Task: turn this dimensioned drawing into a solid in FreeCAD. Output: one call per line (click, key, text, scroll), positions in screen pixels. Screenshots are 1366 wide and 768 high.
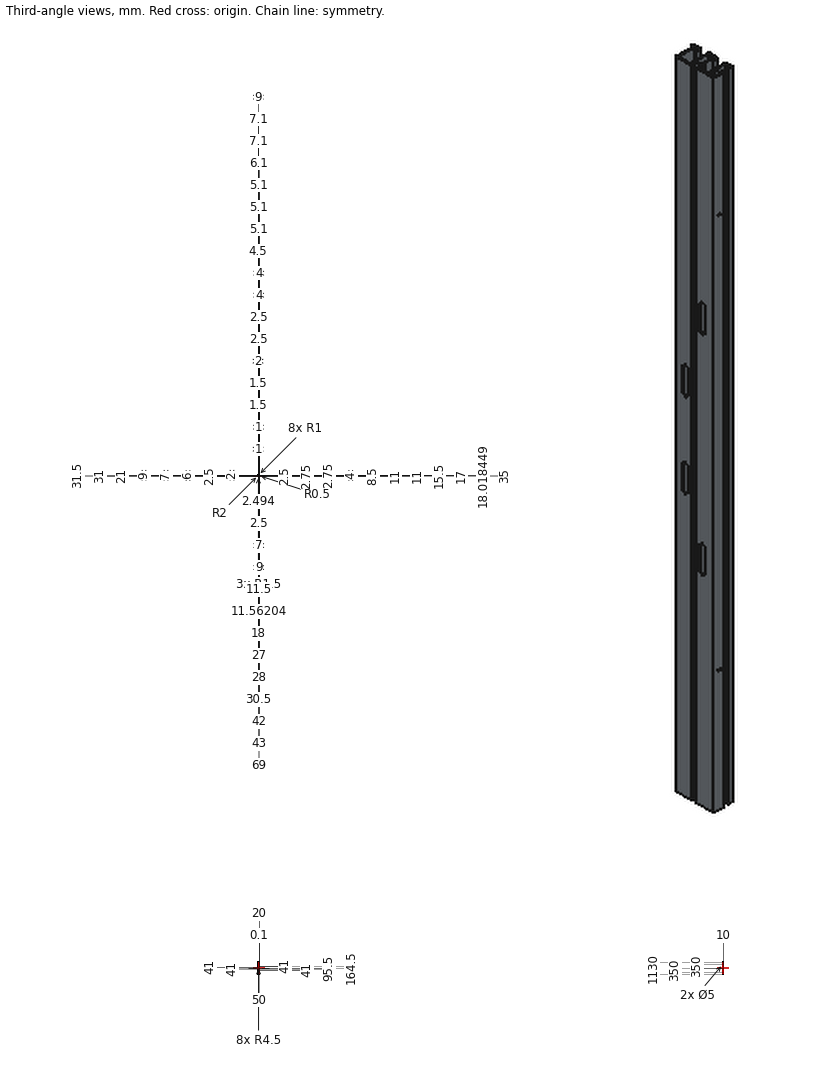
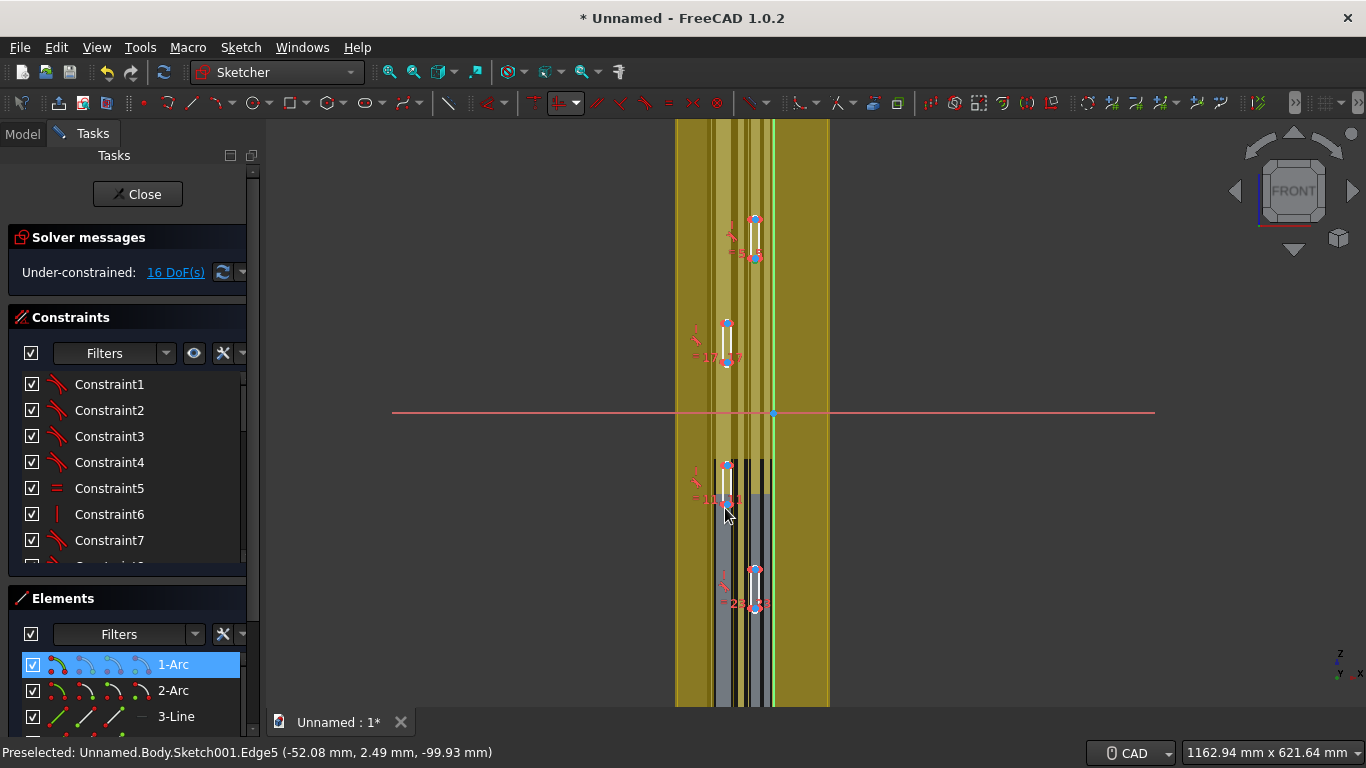
scroll(725, 366, up, 7)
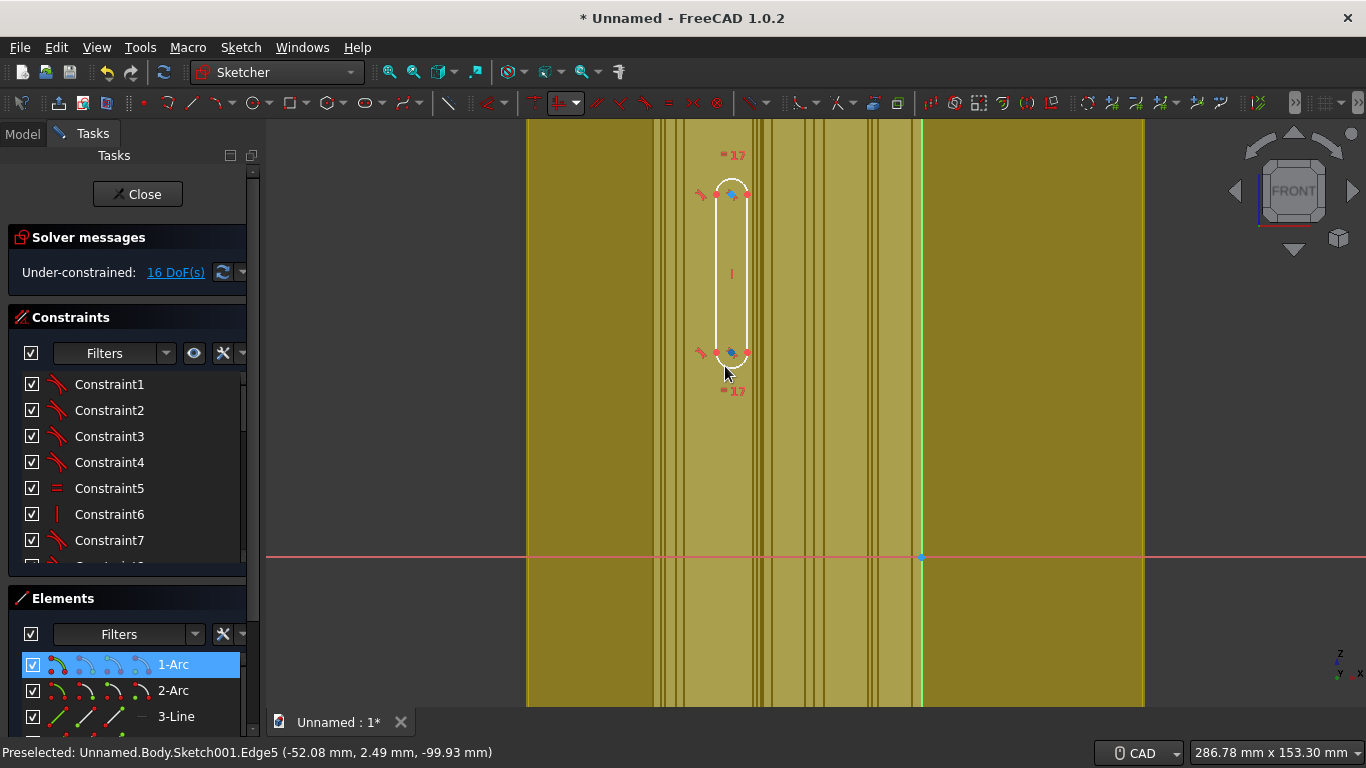
click(723, 365)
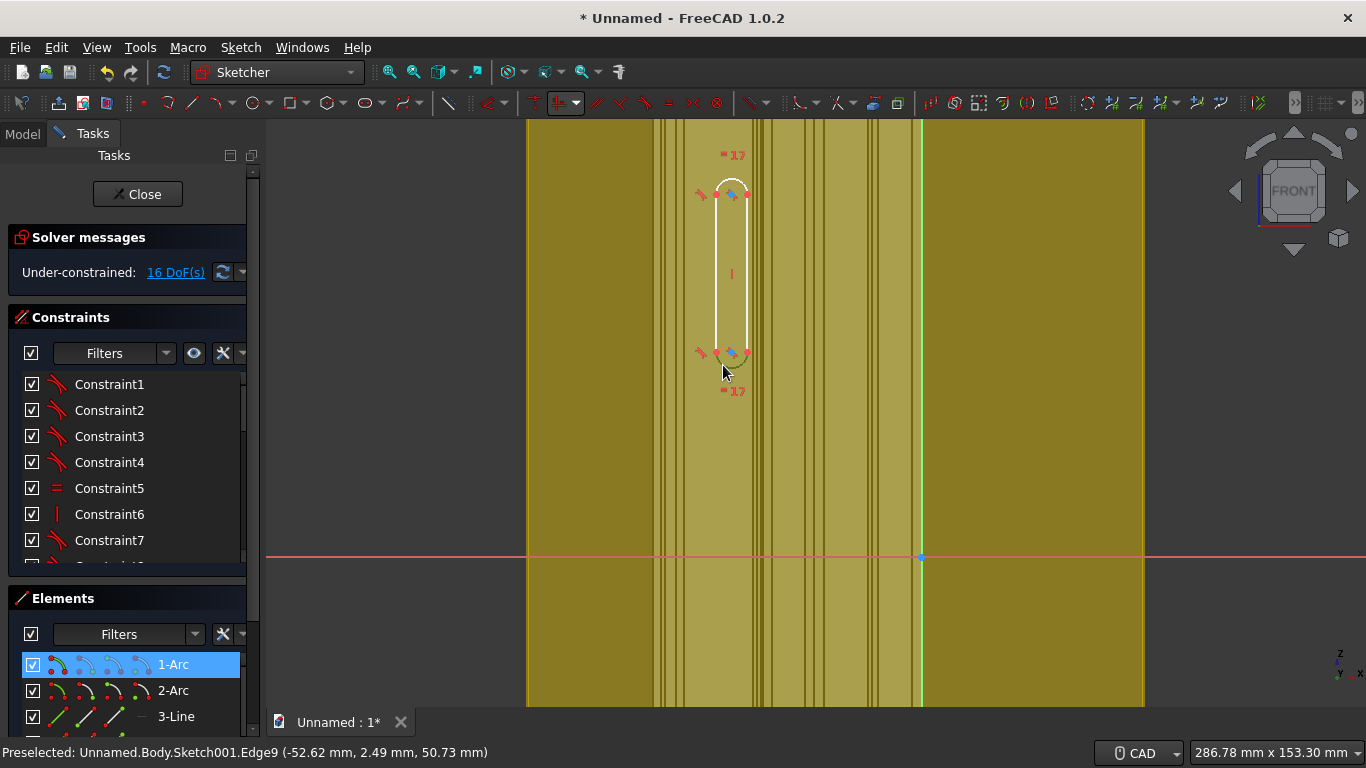
scroll(725, 366, down, 7)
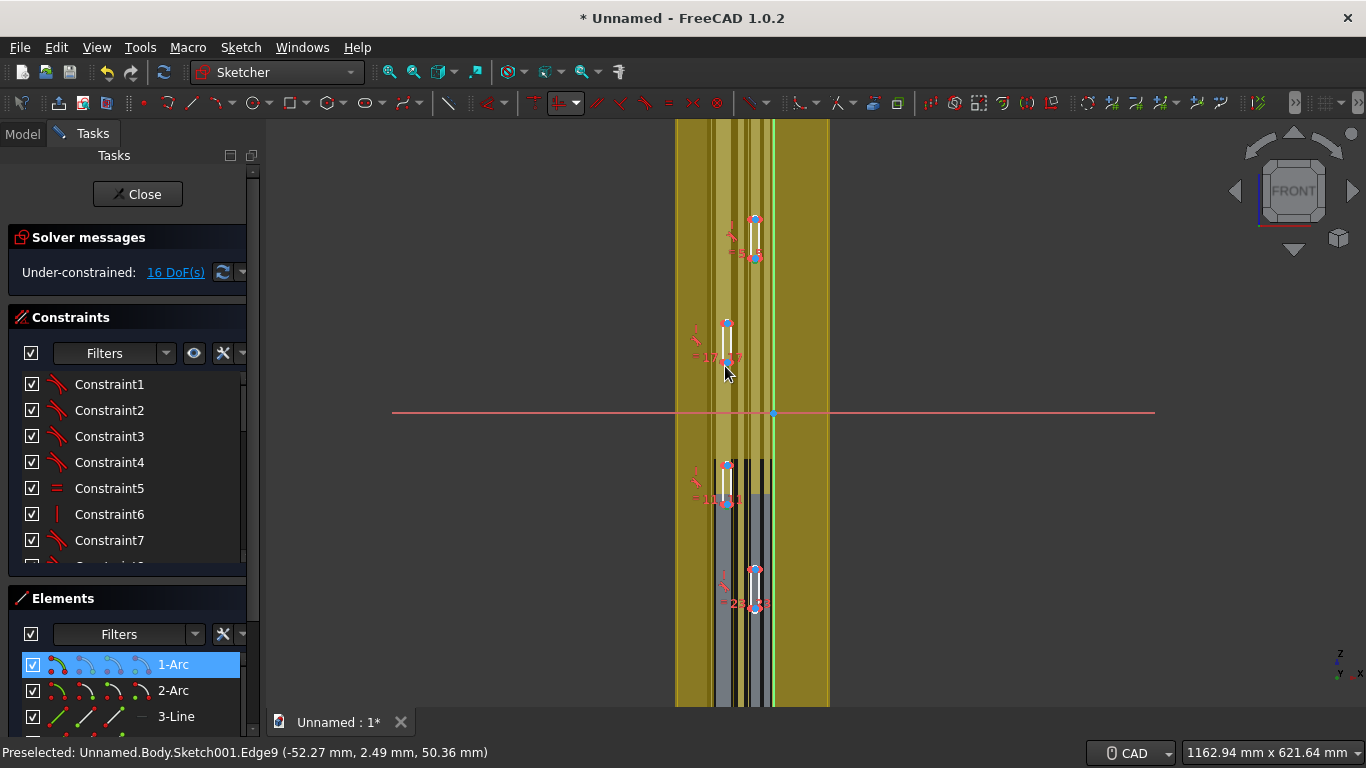
scroll(753, 612, up, 7)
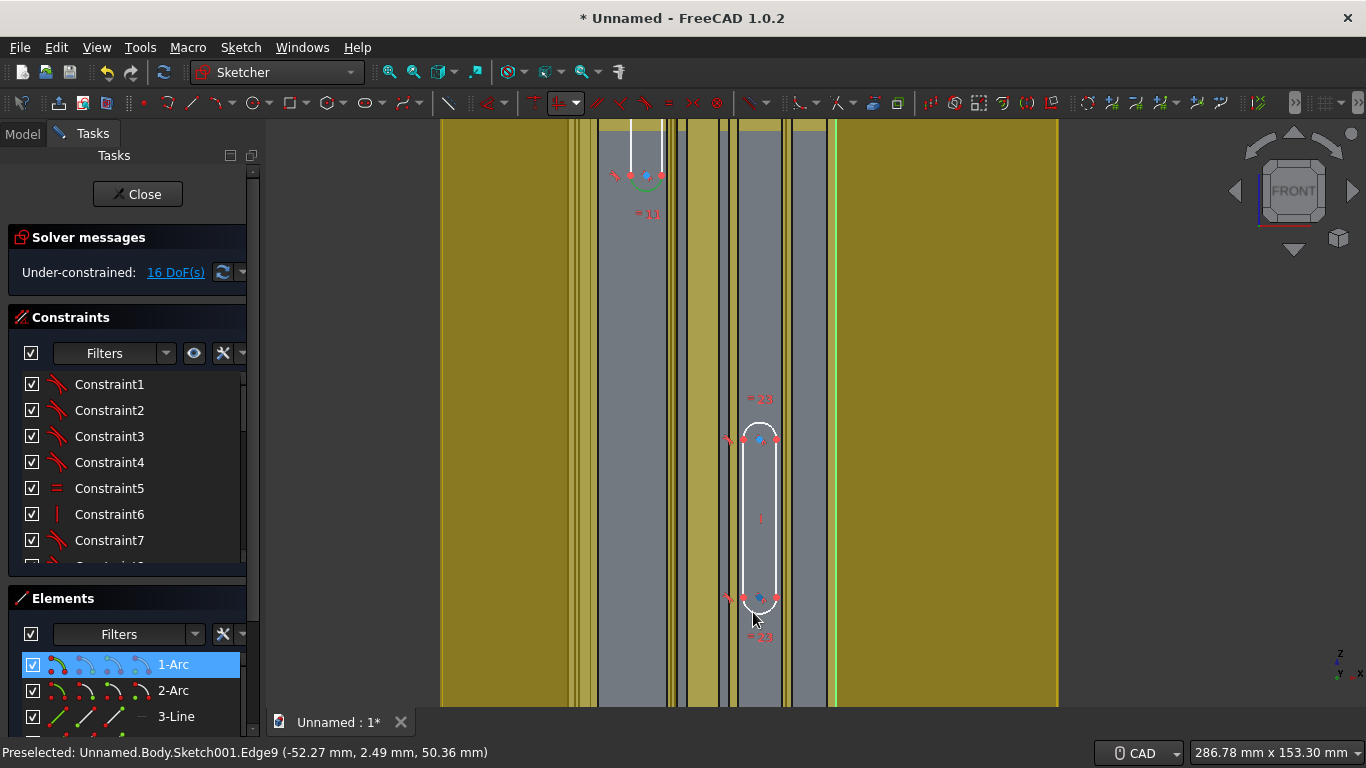
click(750, 611)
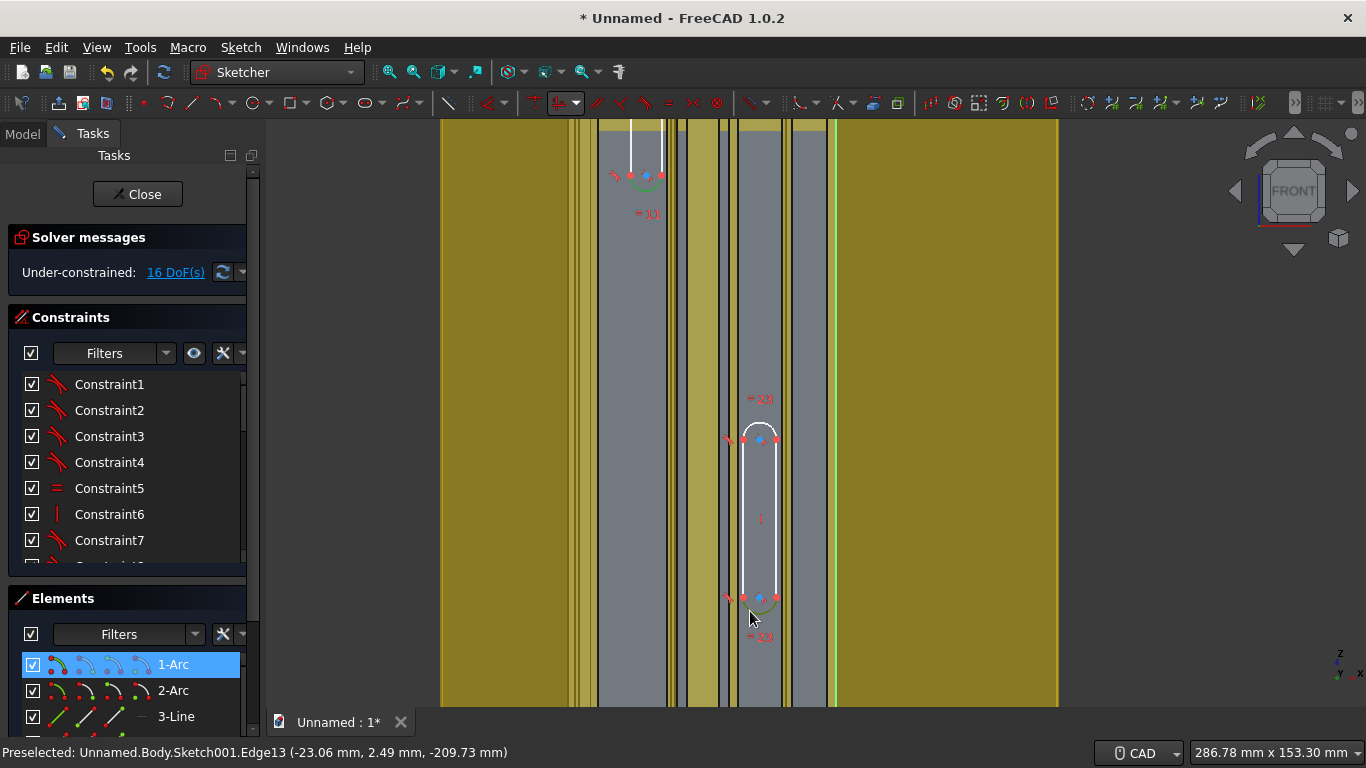
click(670, 104)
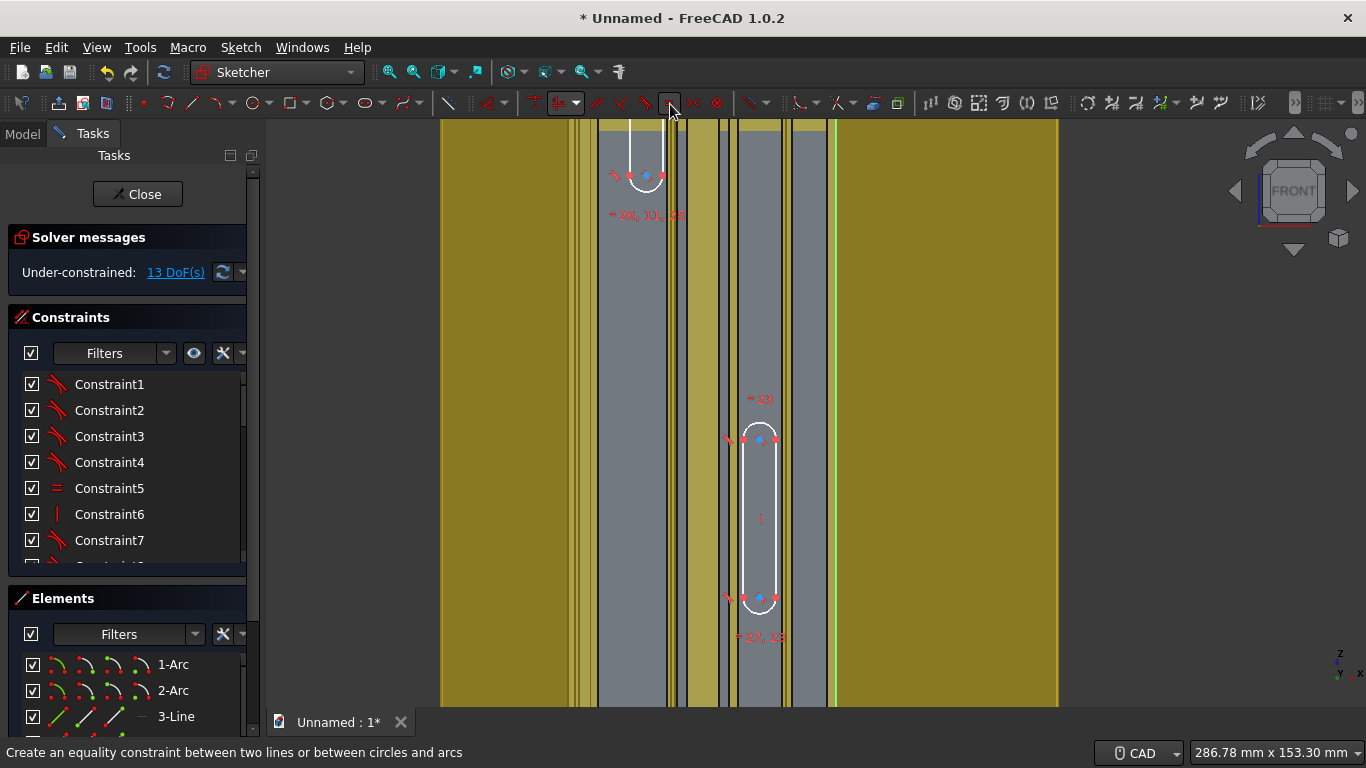
scroll(753, 612, down, 7)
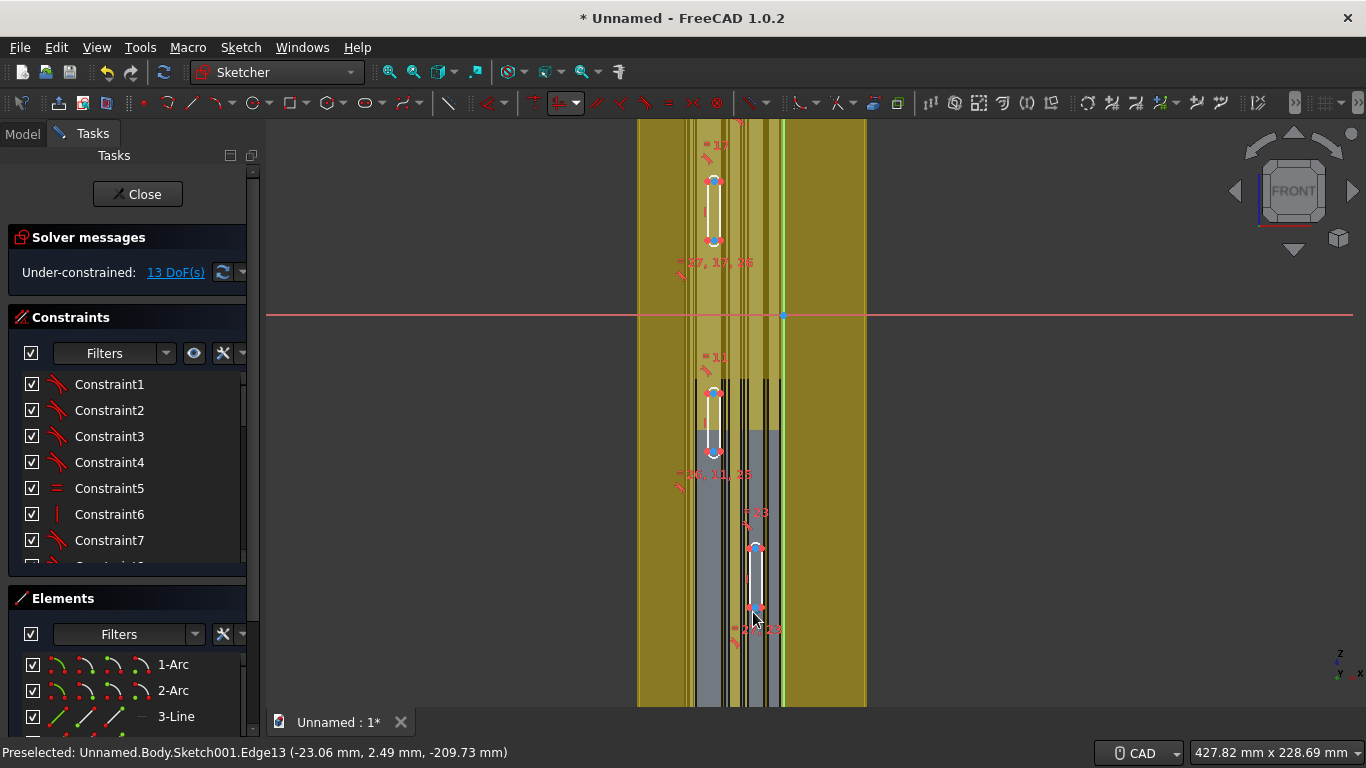
scroll(727, 466, up, 6)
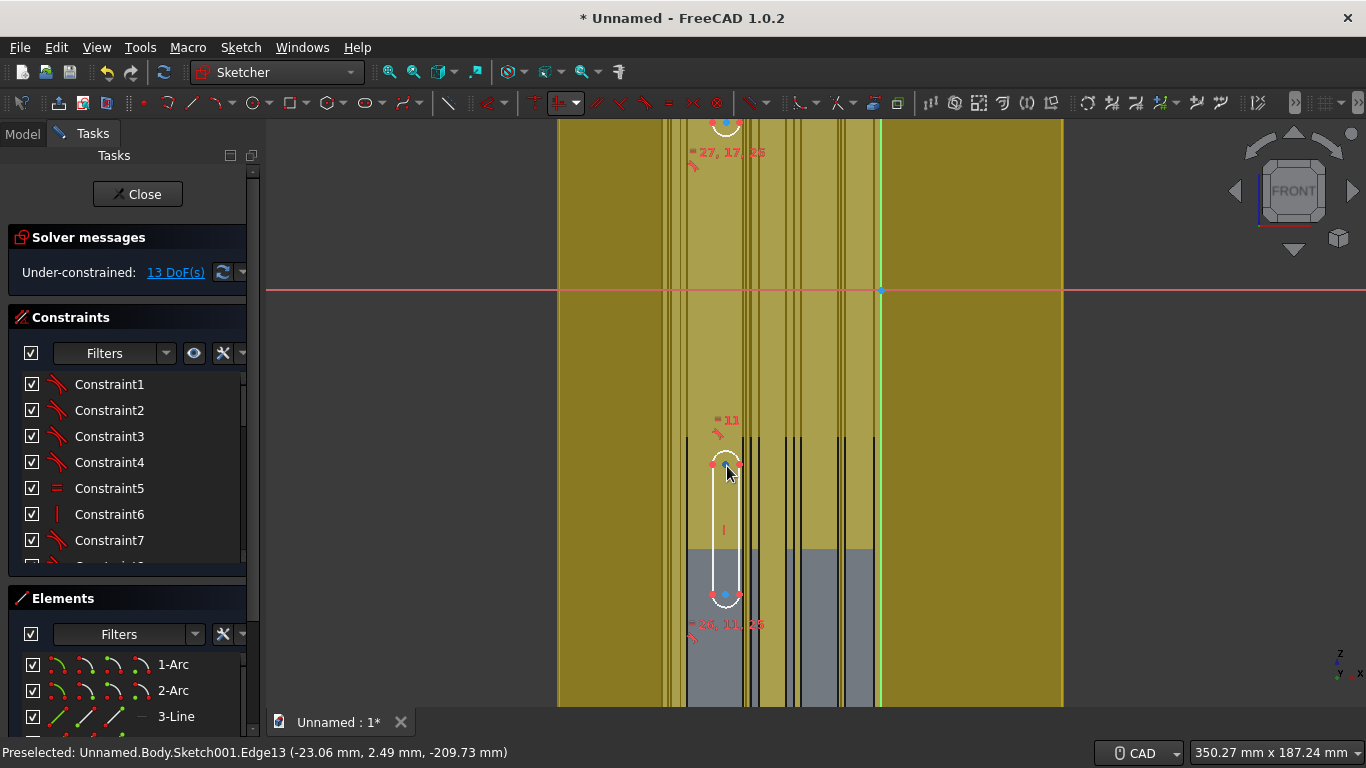
click(726, 465)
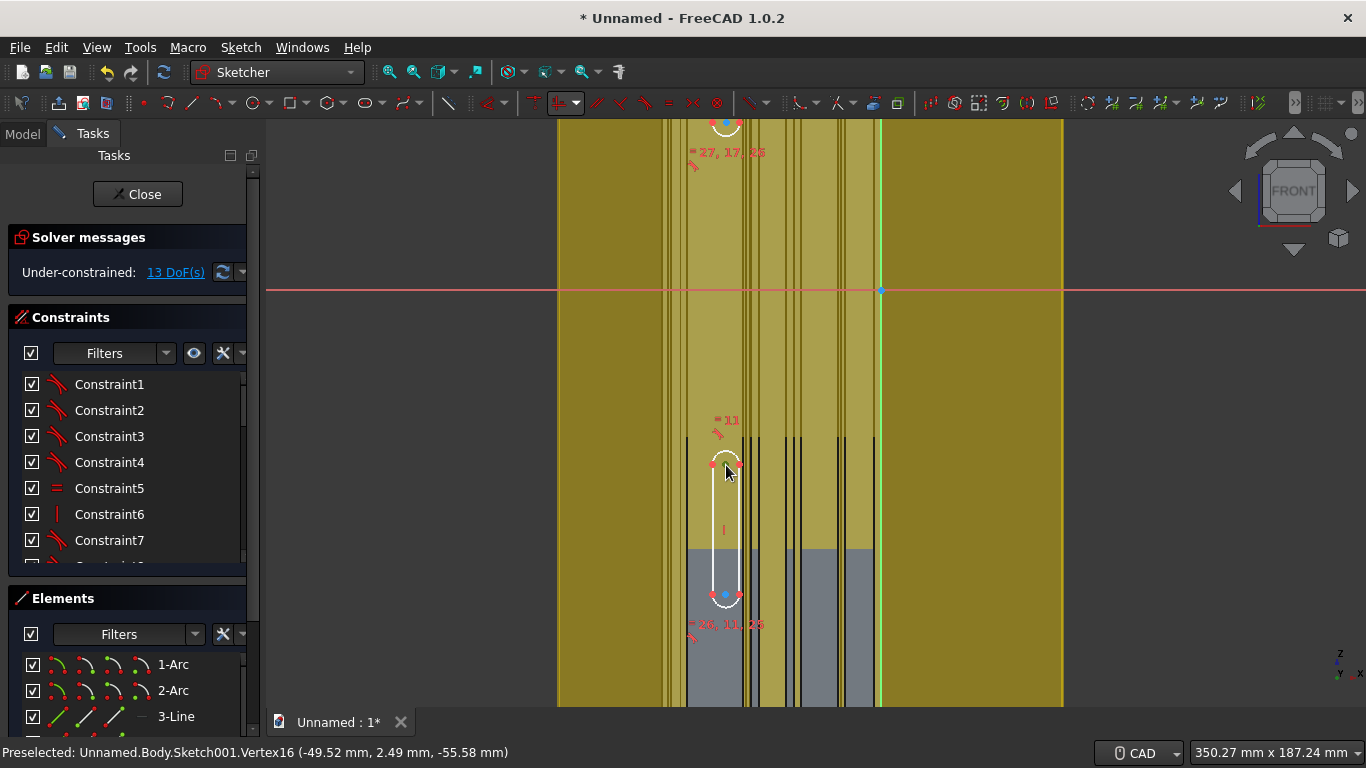
scroll(727, 466, down, 6)